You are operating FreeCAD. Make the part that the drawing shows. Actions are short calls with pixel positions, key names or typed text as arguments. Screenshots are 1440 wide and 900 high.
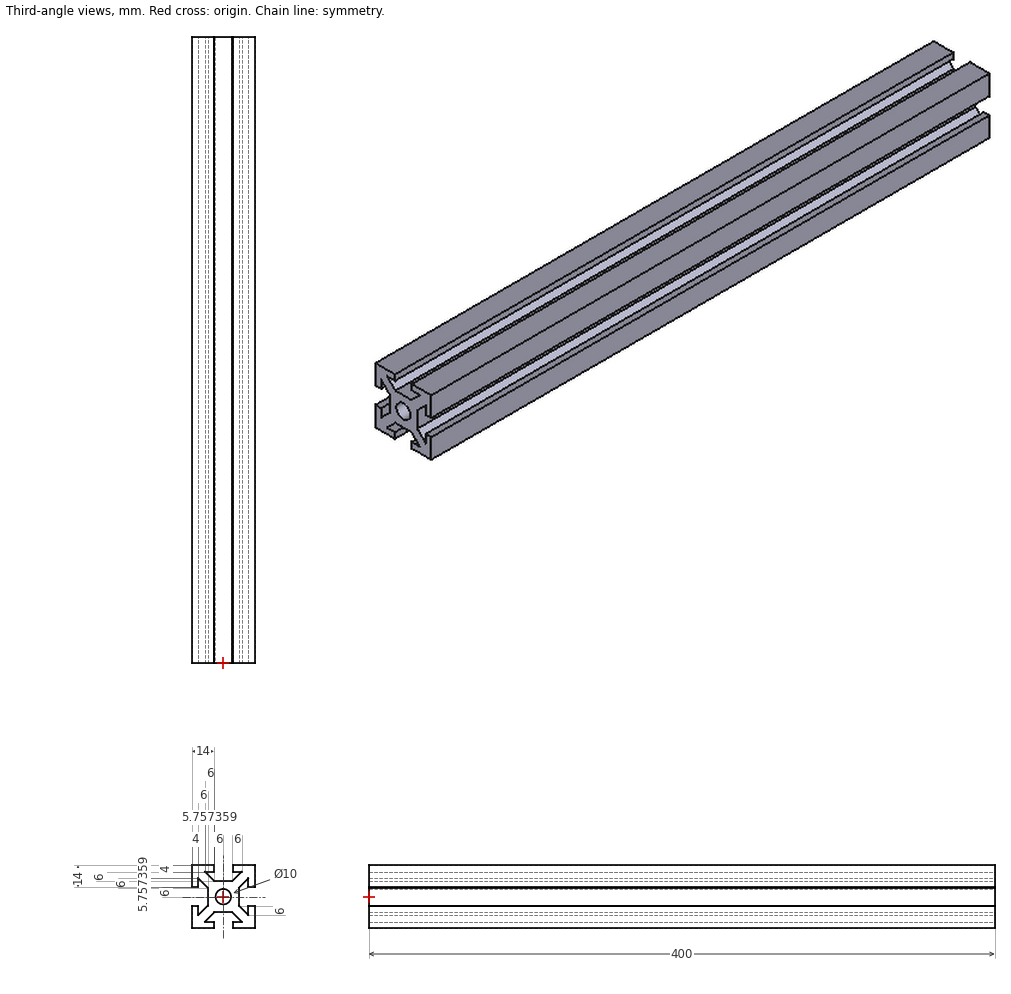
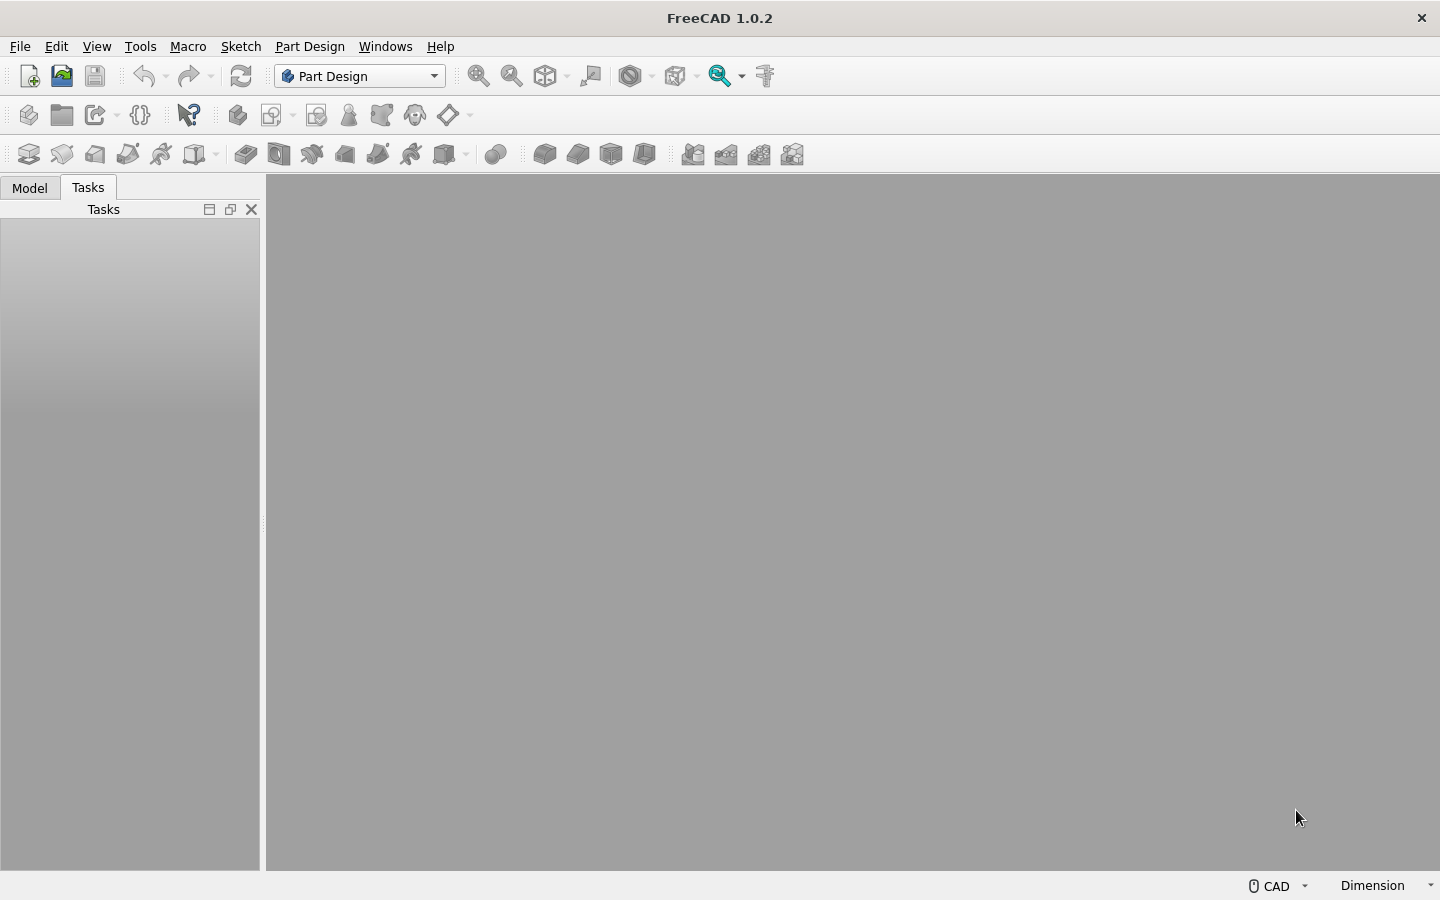
key(ctrl+n)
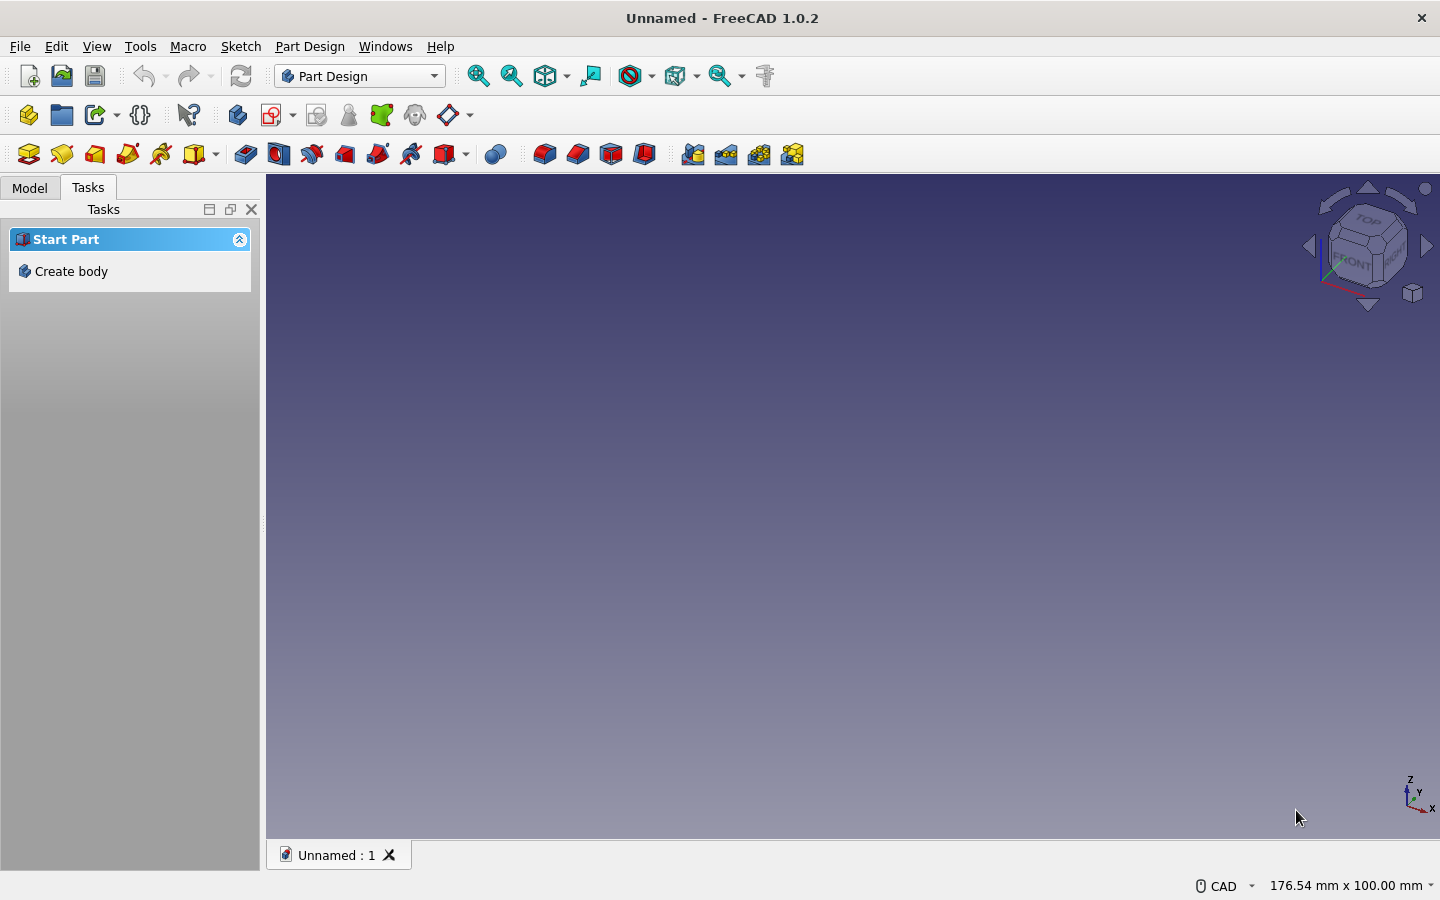
click(270, 116)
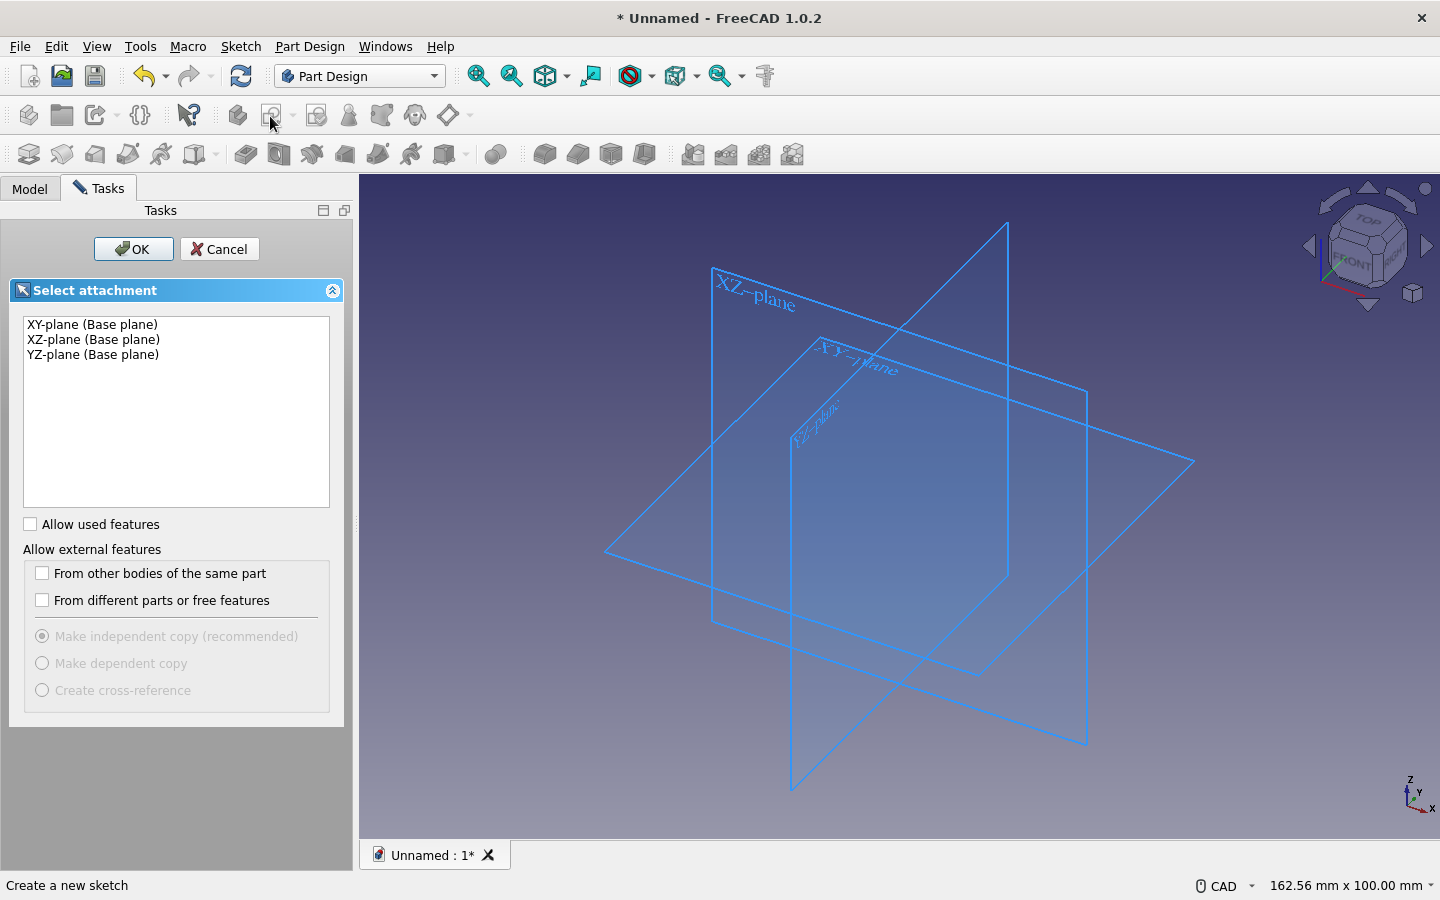
click(84, 340)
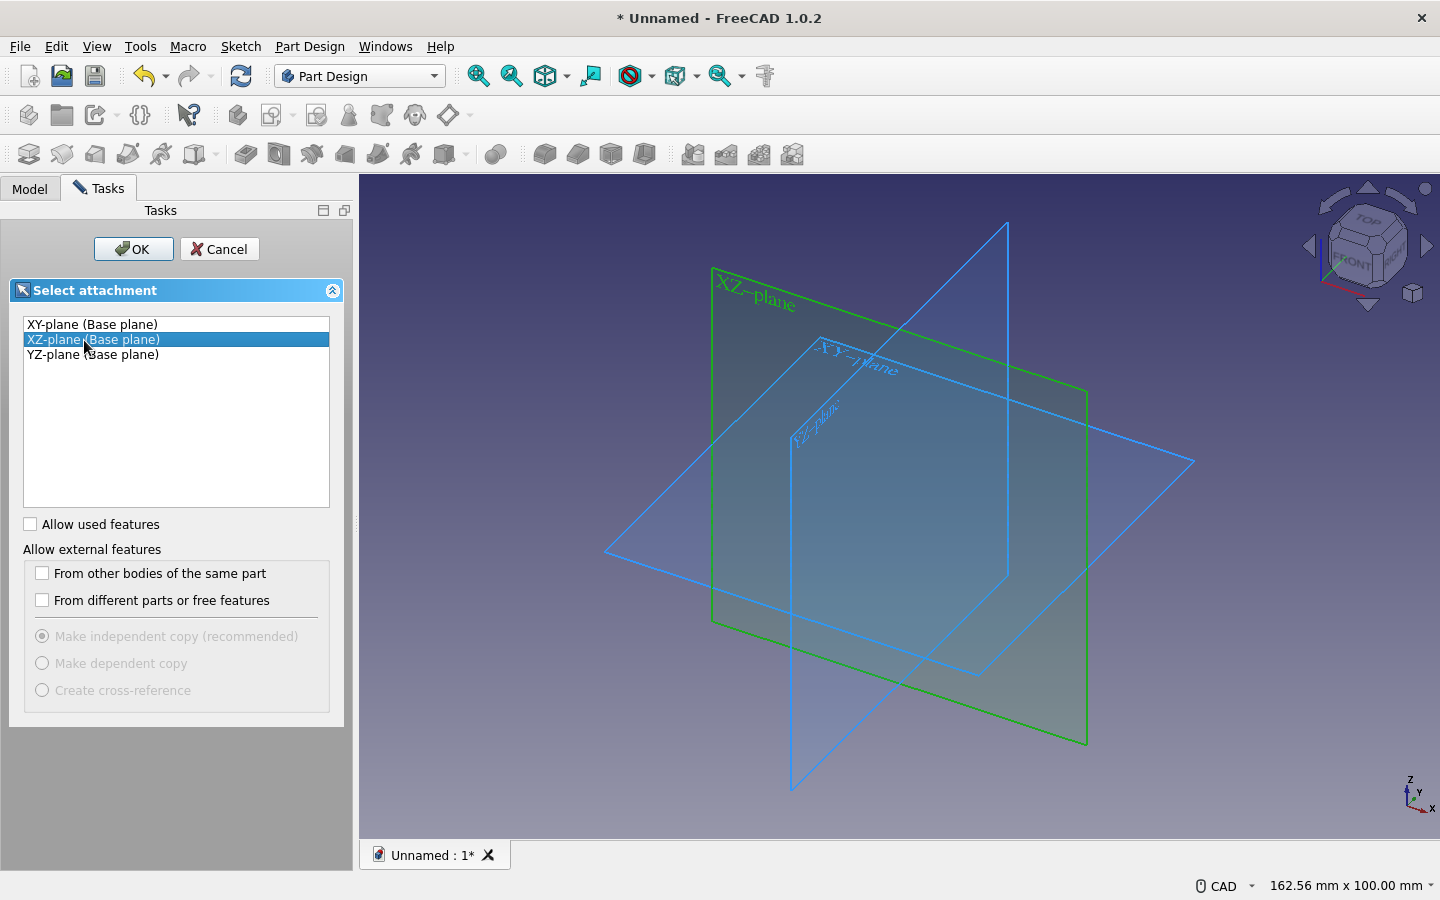
click(134, 249)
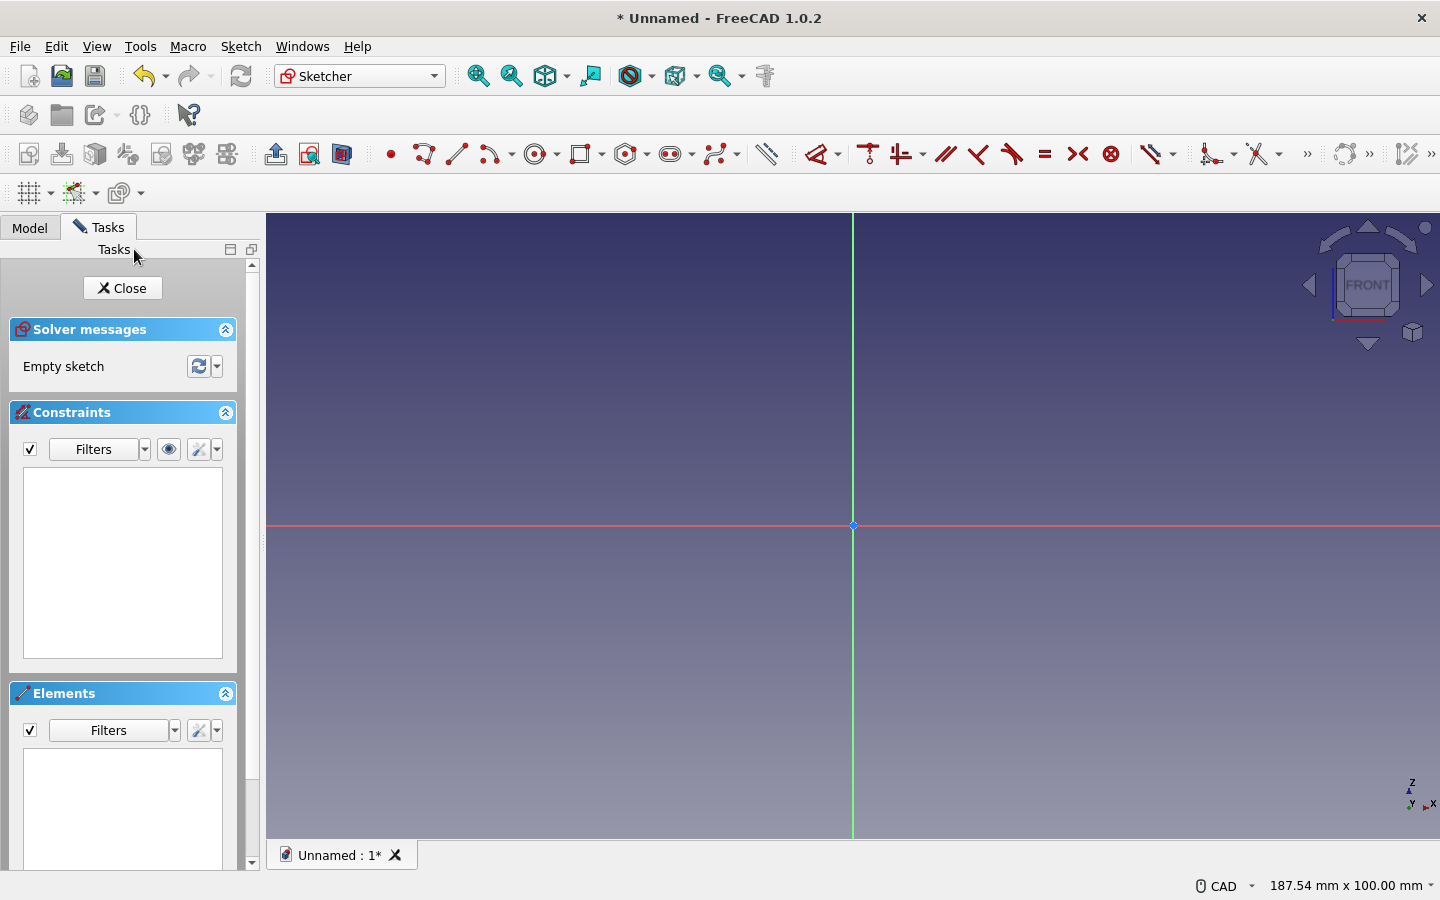
scroll(992, 526, up, 2)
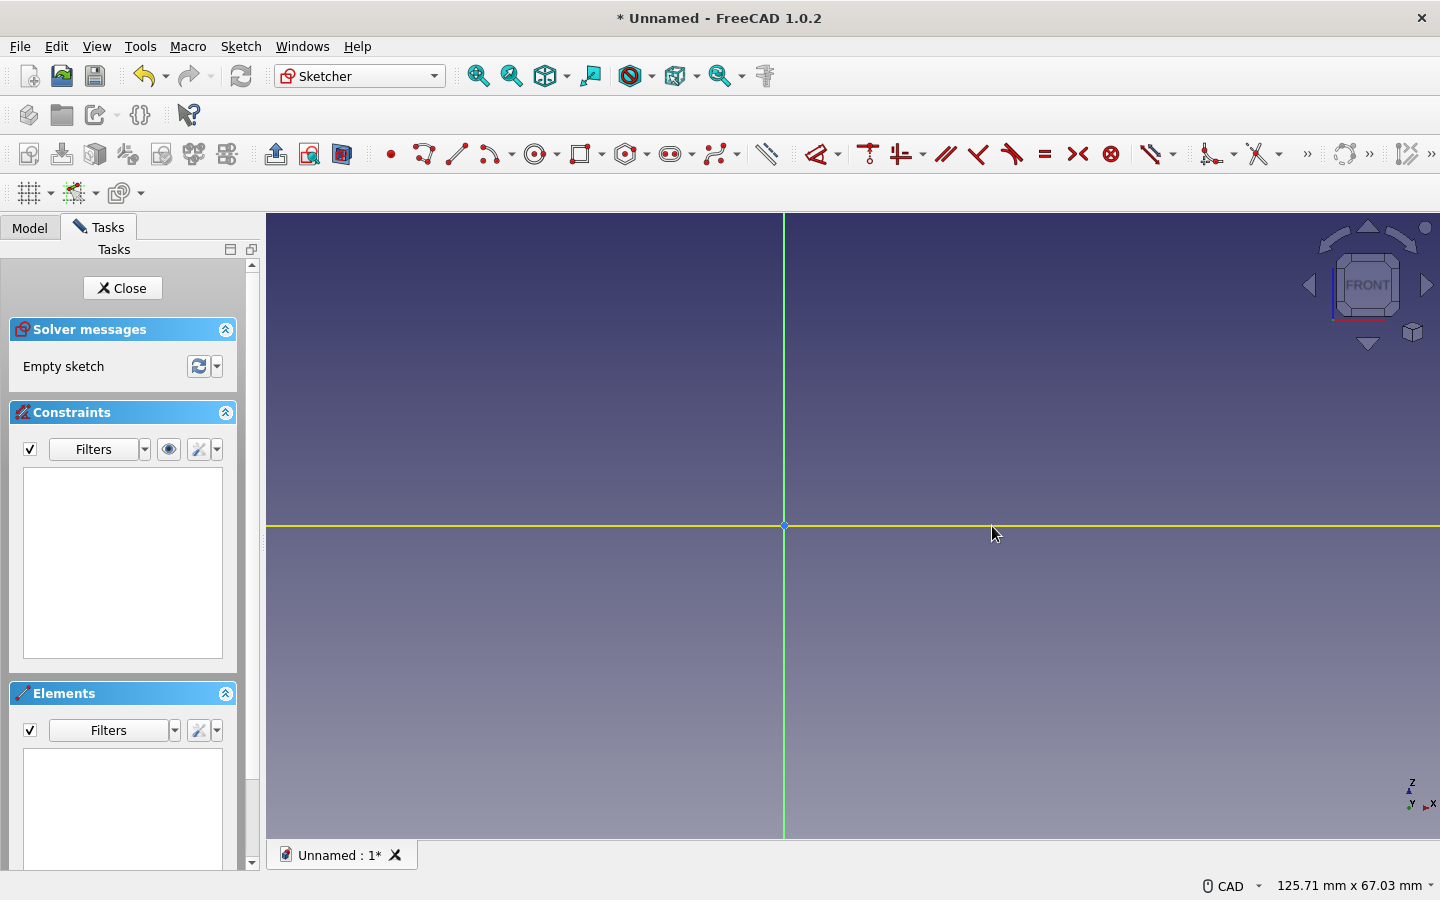
click(424, 154)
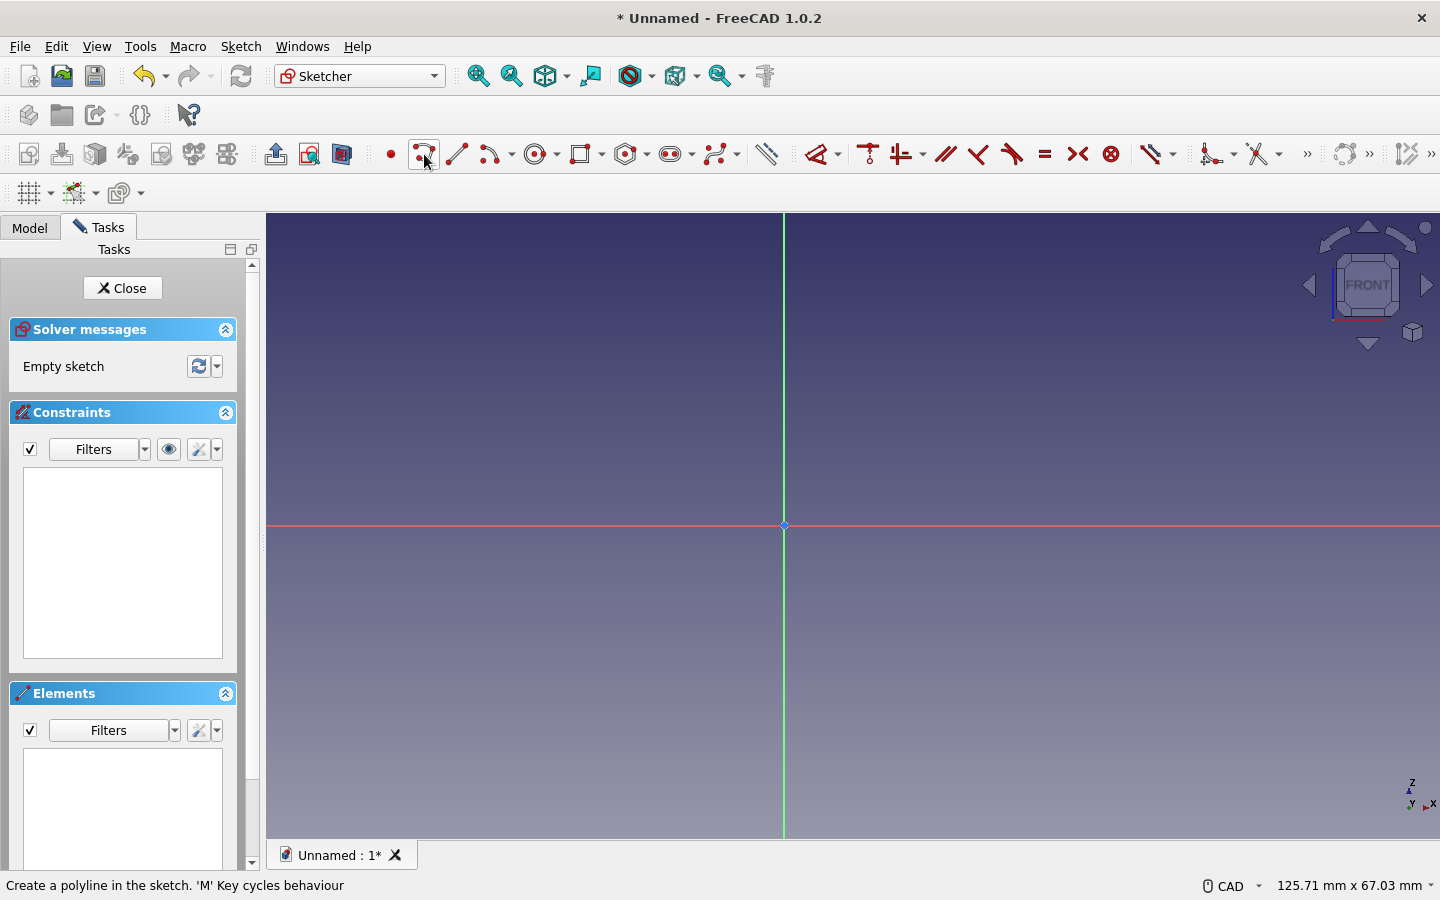
click(691, 580)
click(691, 472)
click(635, 416)
click(635, 470)
click(598, 470)
click(598, 339)
click(728, 339)
click(728, 376)
click(675, 376)
click(731, 432)
click(838, 432)
click(894, 376)
click(840, 376)
click(840, 339)
click(971, 339)
click(971, 470)
click(934, 470)
click(934, 416)
click(878, 472)
click(878, 580)
click(934, 636)
click(934, 582)
click(971, 582)
click(971, 713)
click(840, 713)
click(840, 675)
click(894, 675)
click(838, 619)
click(731, 619)
click(675, 675)
click(728, 675)
click(728, 713)
click(598, 713)
click(598, 582)
click(635, 582)
click(635, 636)
click(691, 581)